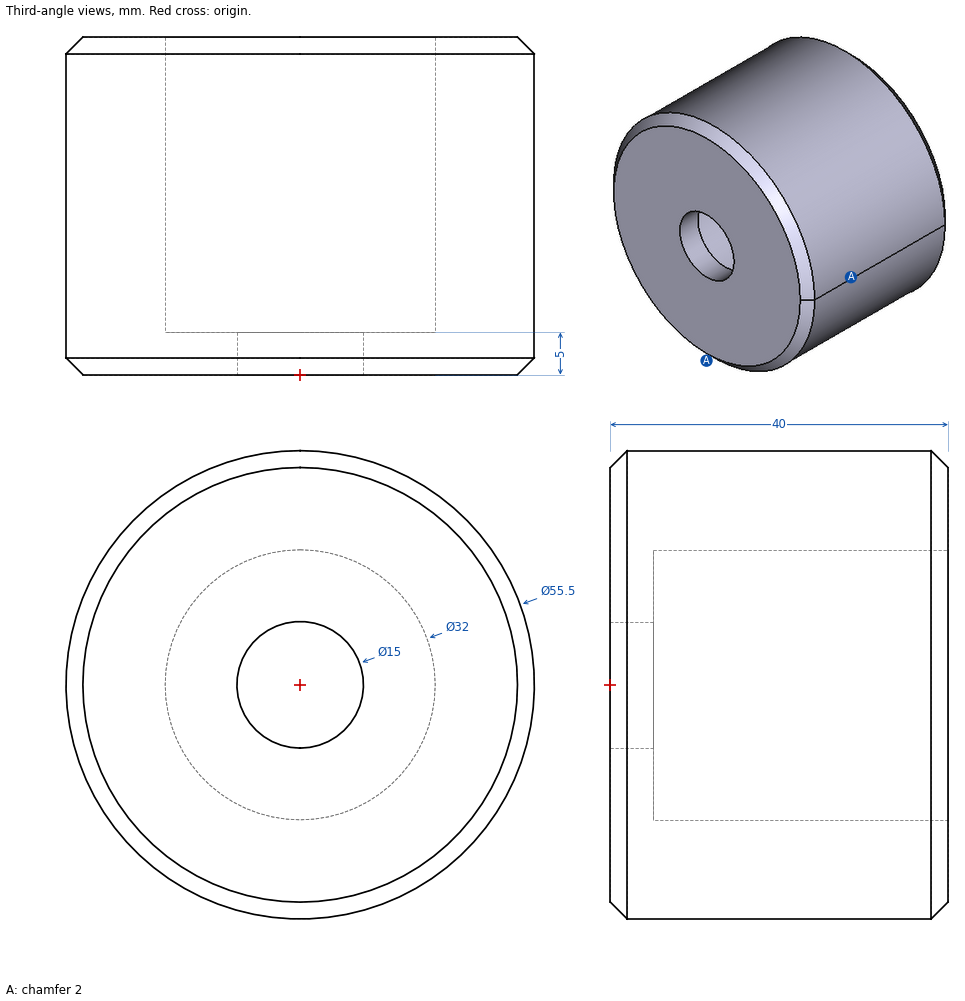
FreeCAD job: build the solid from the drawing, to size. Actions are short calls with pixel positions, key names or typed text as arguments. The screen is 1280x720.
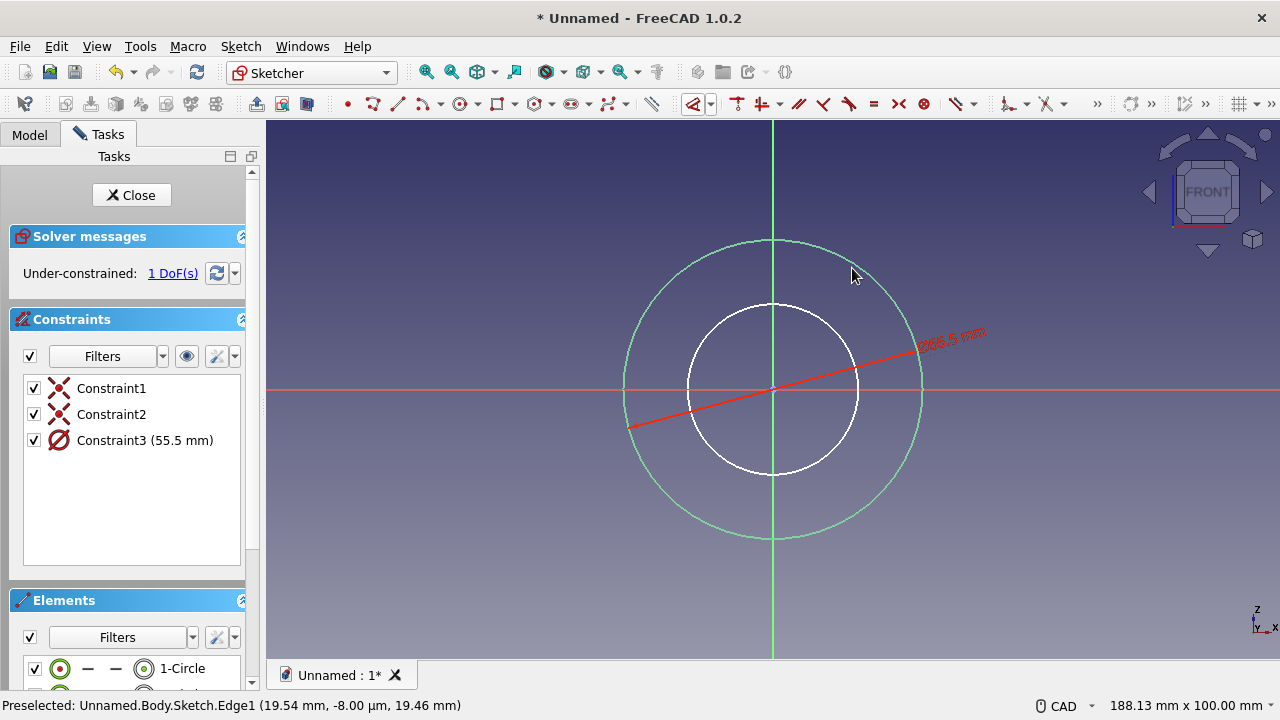
click(833, 329)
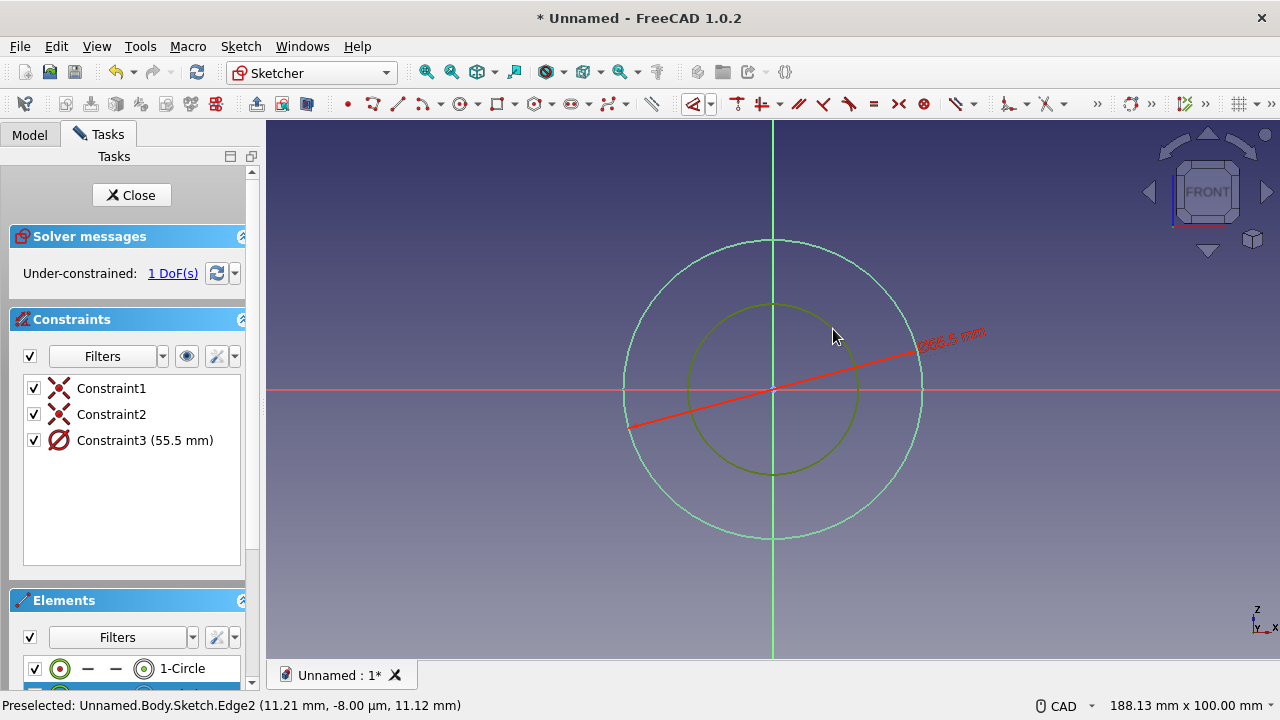
click(710, 104)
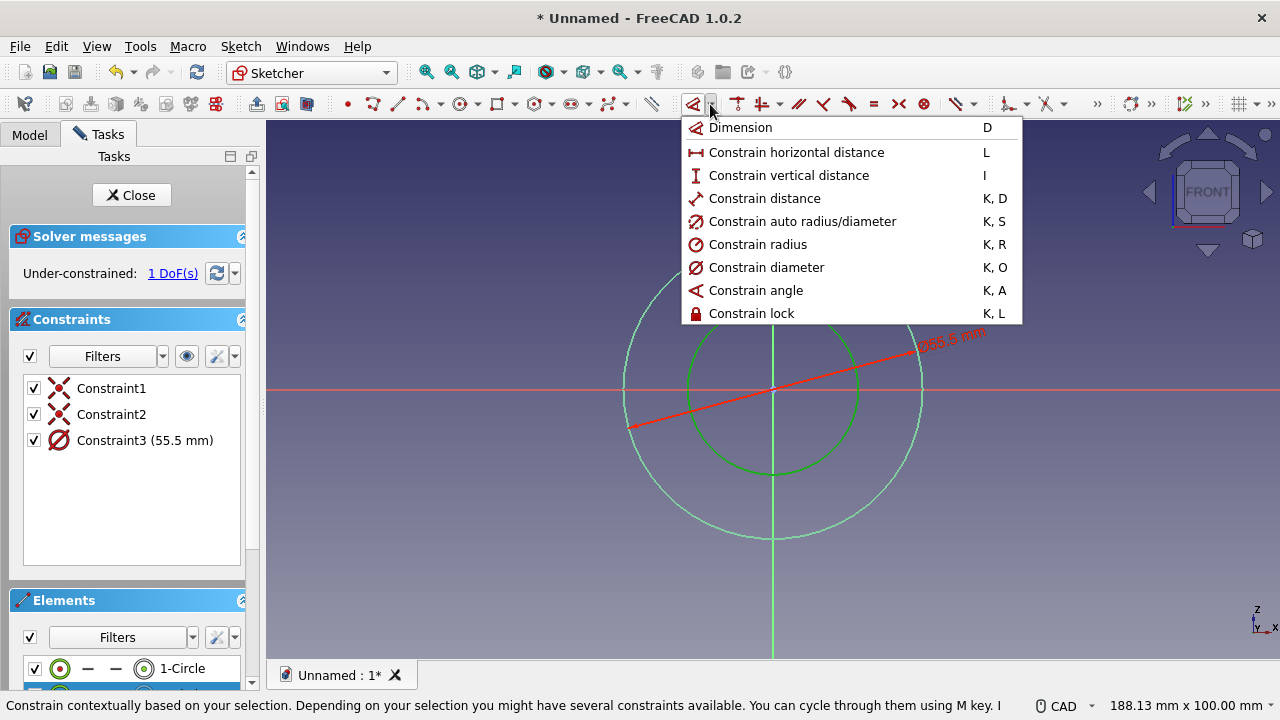
click(852, 268)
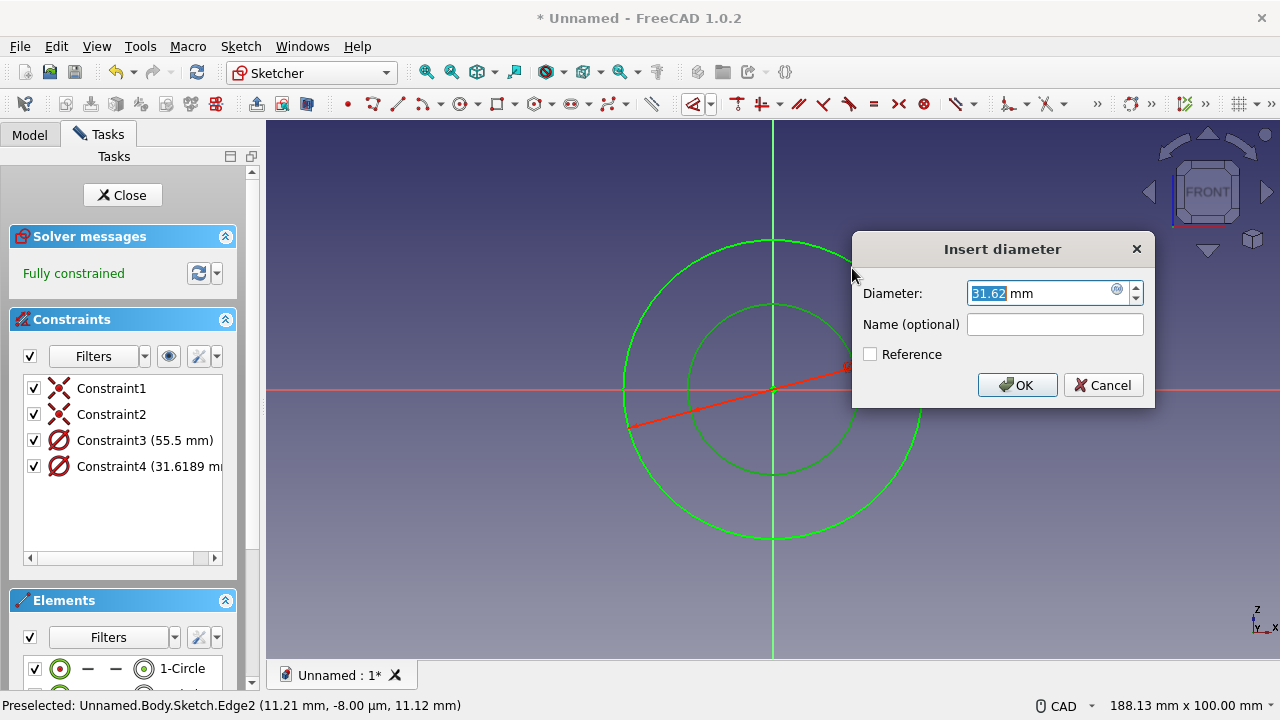
text(32)
key(Return)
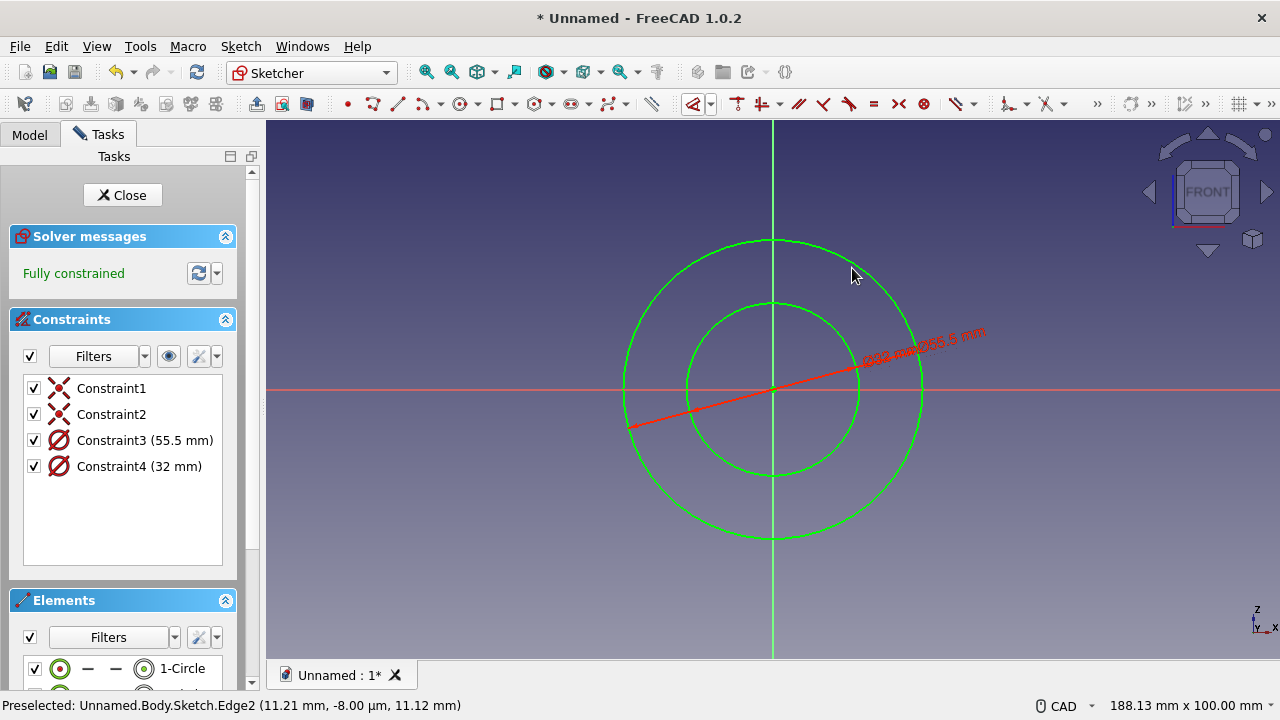
click(123, 195)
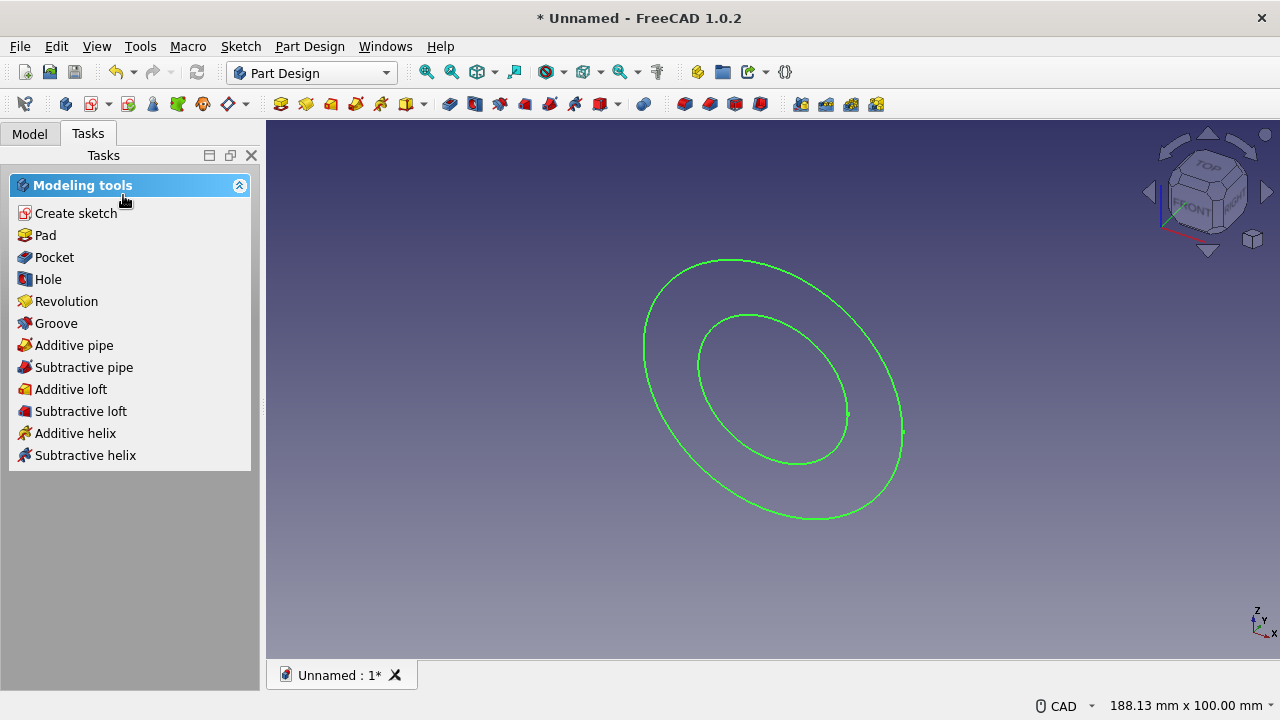
click(281, 104)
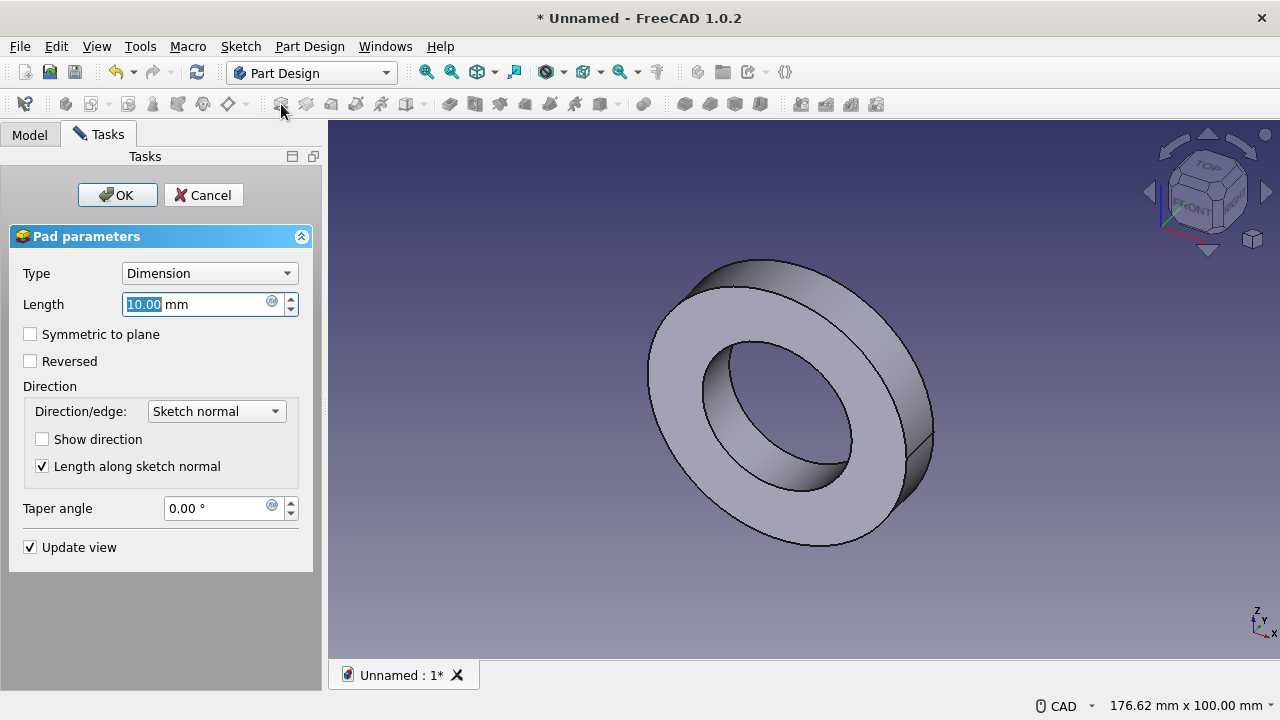
text(40)
key(Tab)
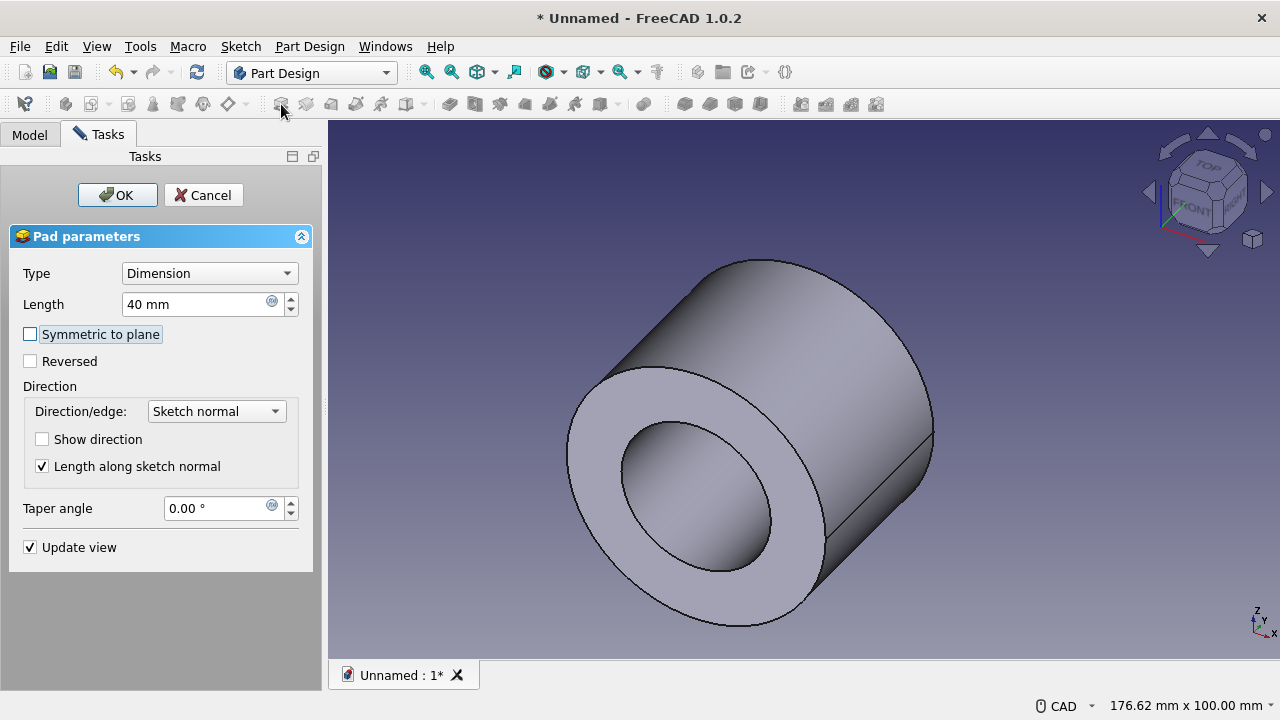
click(31, 361)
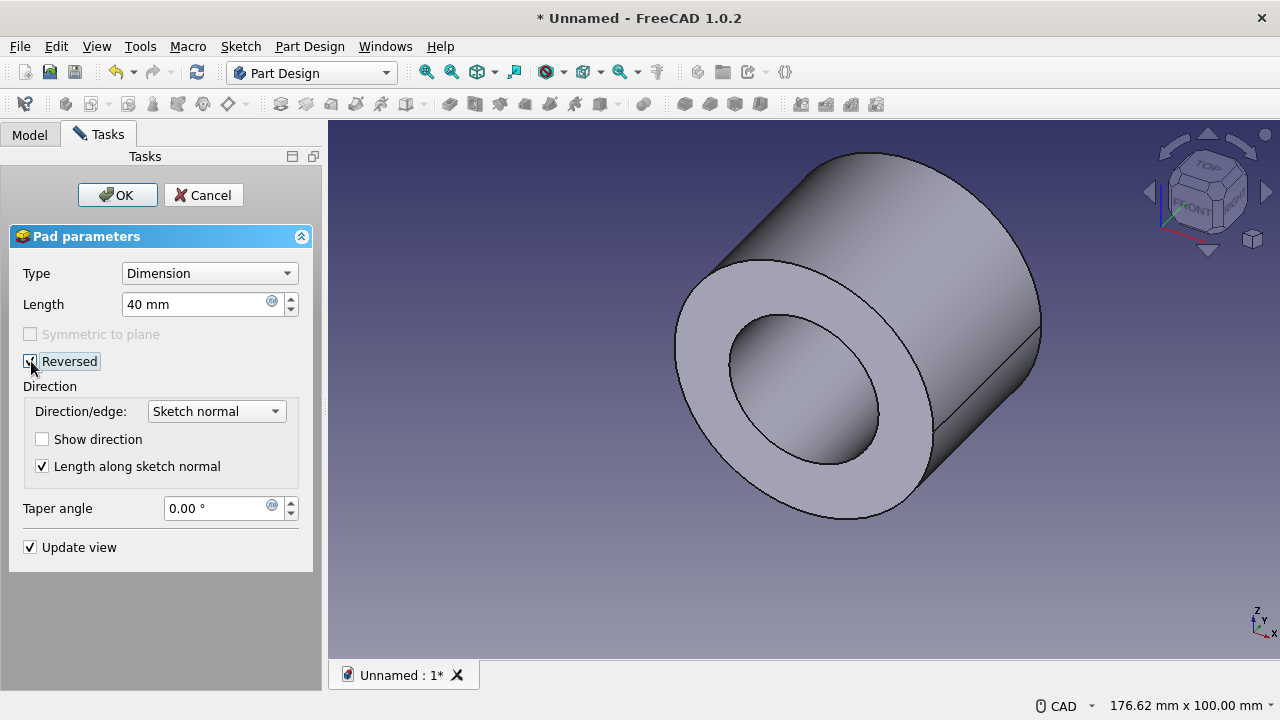
click(118, 195)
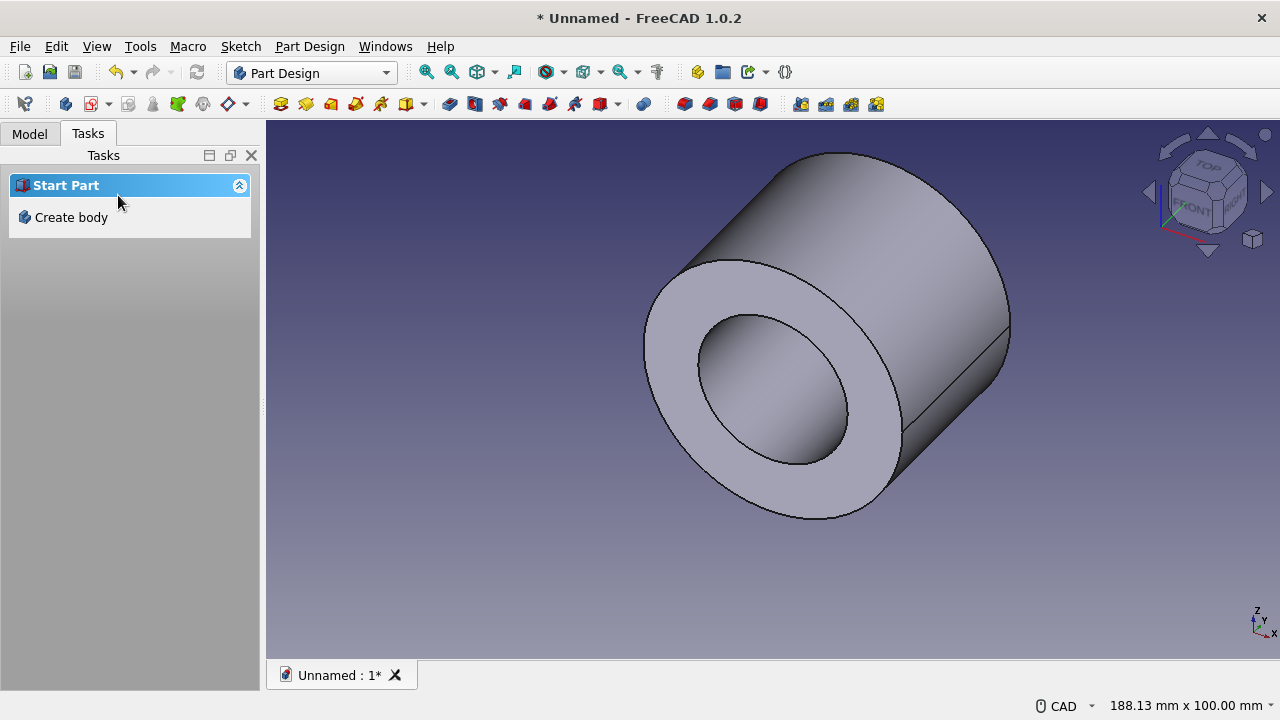
click(427, 72)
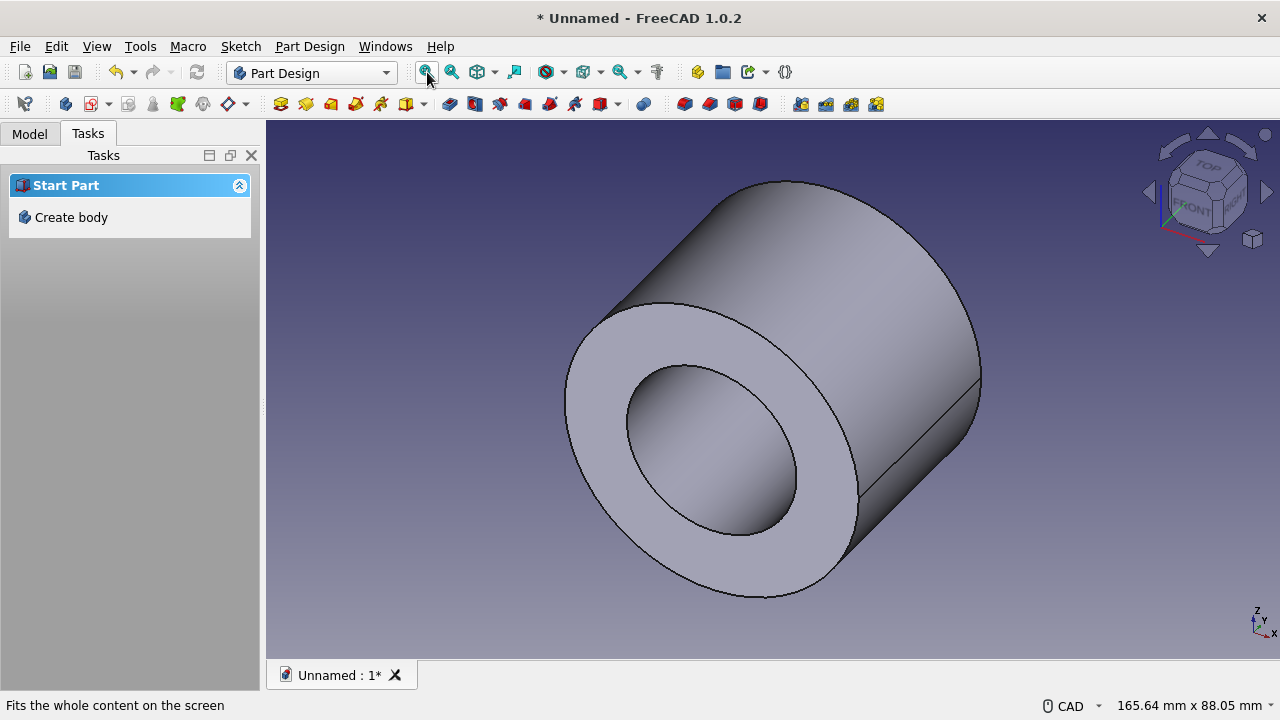
click(593, 328)